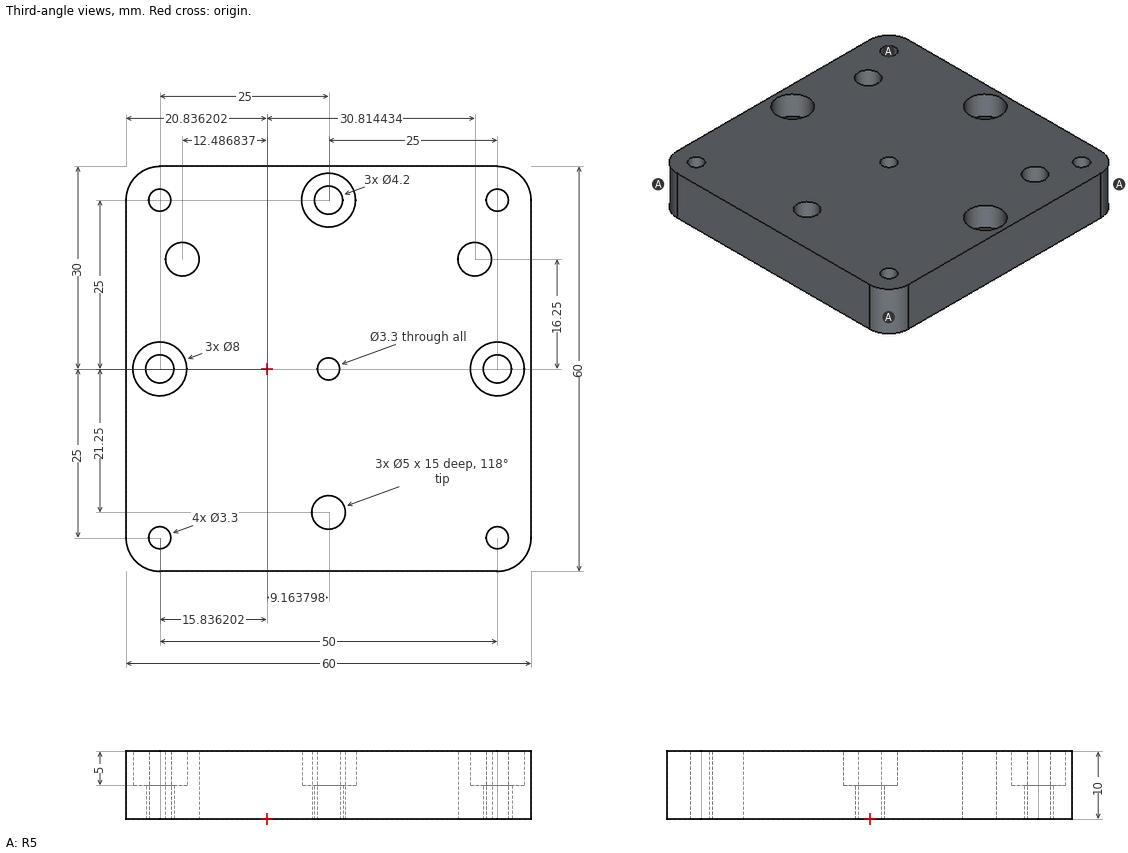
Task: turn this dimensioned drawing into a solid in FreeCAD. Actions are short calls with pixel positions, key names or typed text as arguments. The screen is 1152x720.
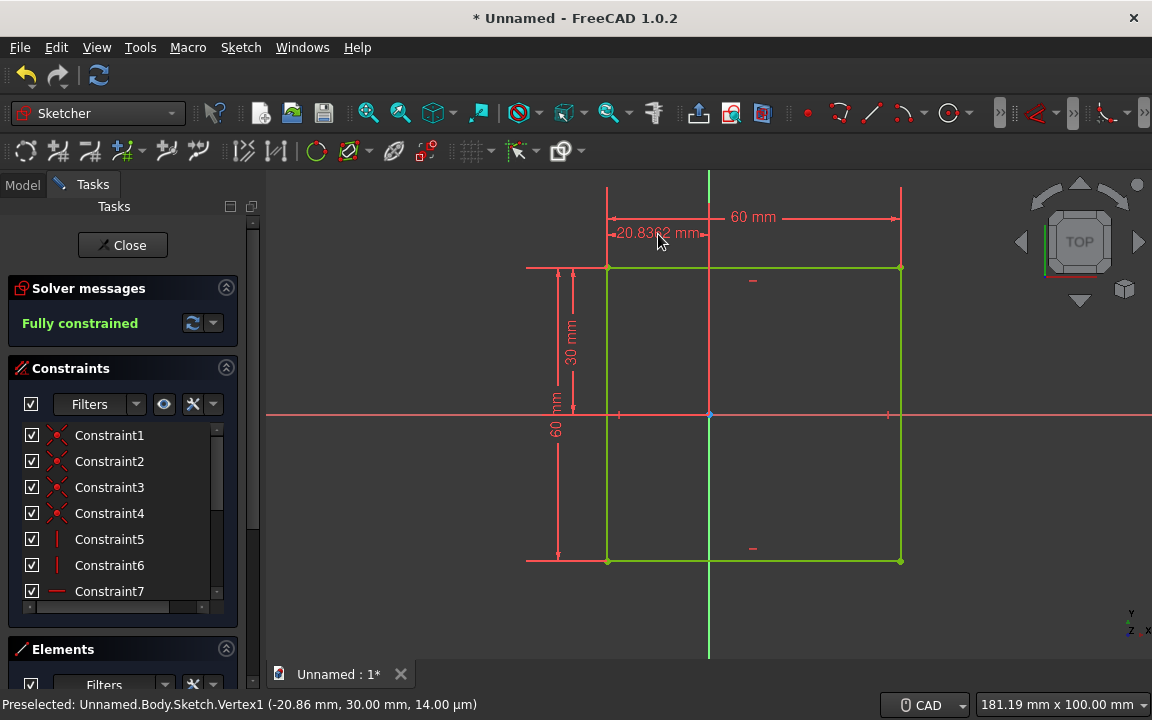
click(123, 245)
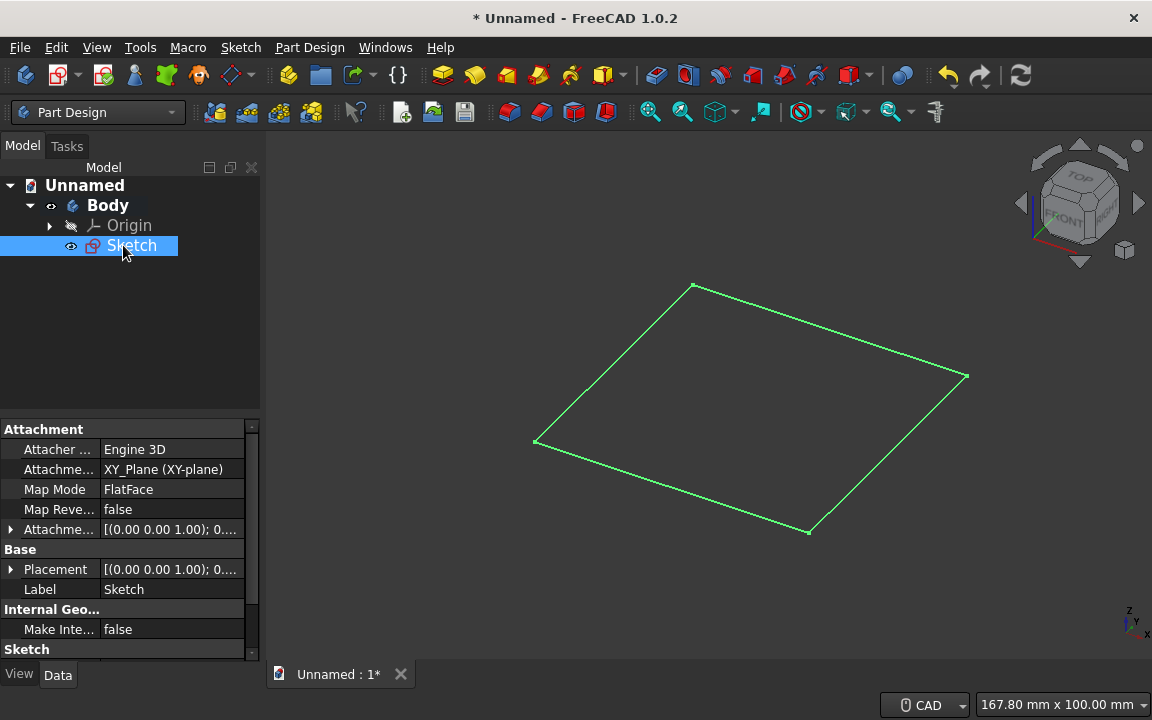
click(444, 76)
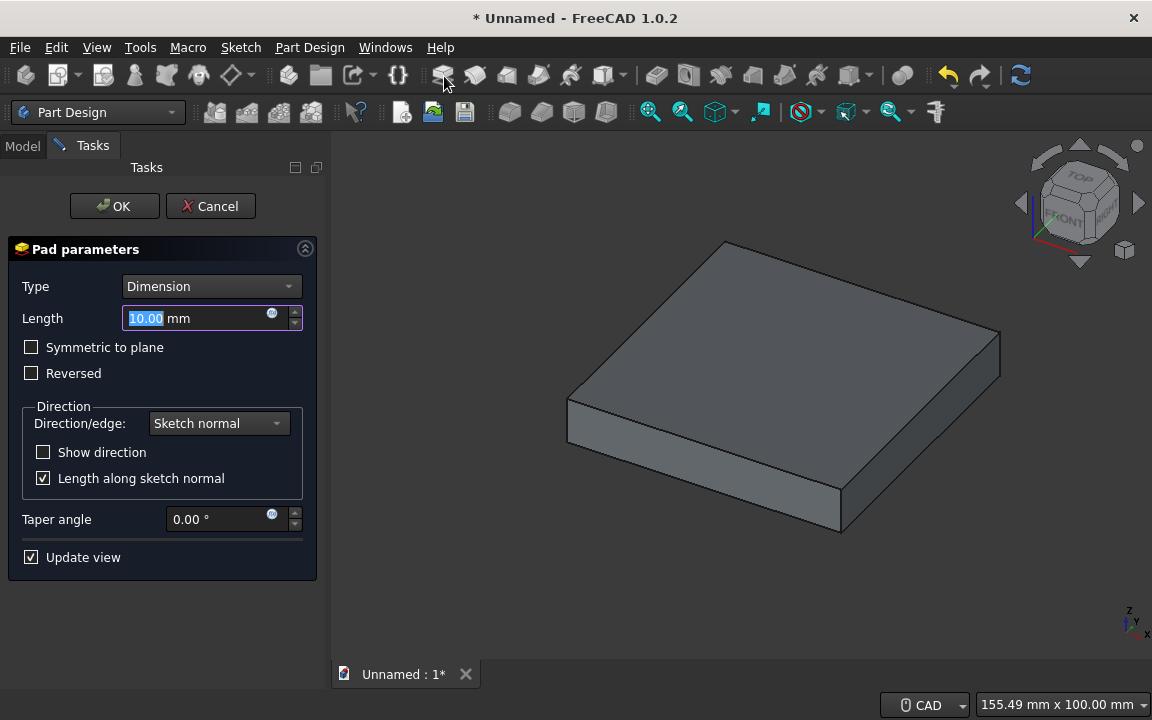
text(10)
key(Tab)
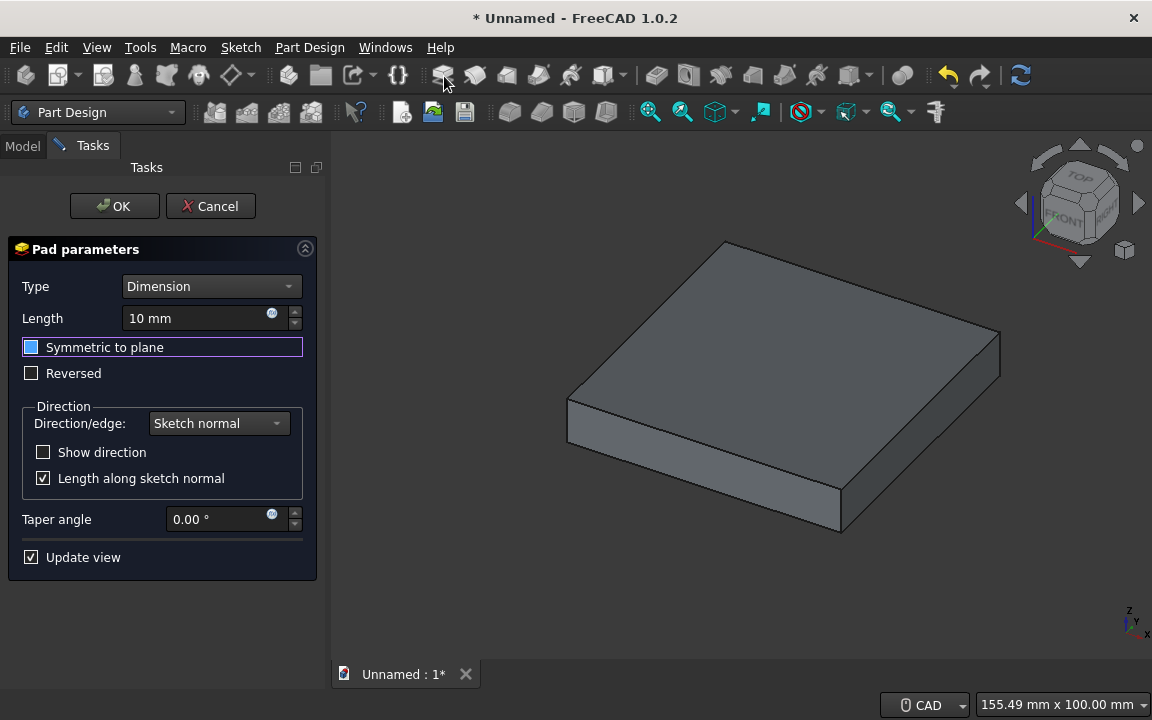
click(115, 206)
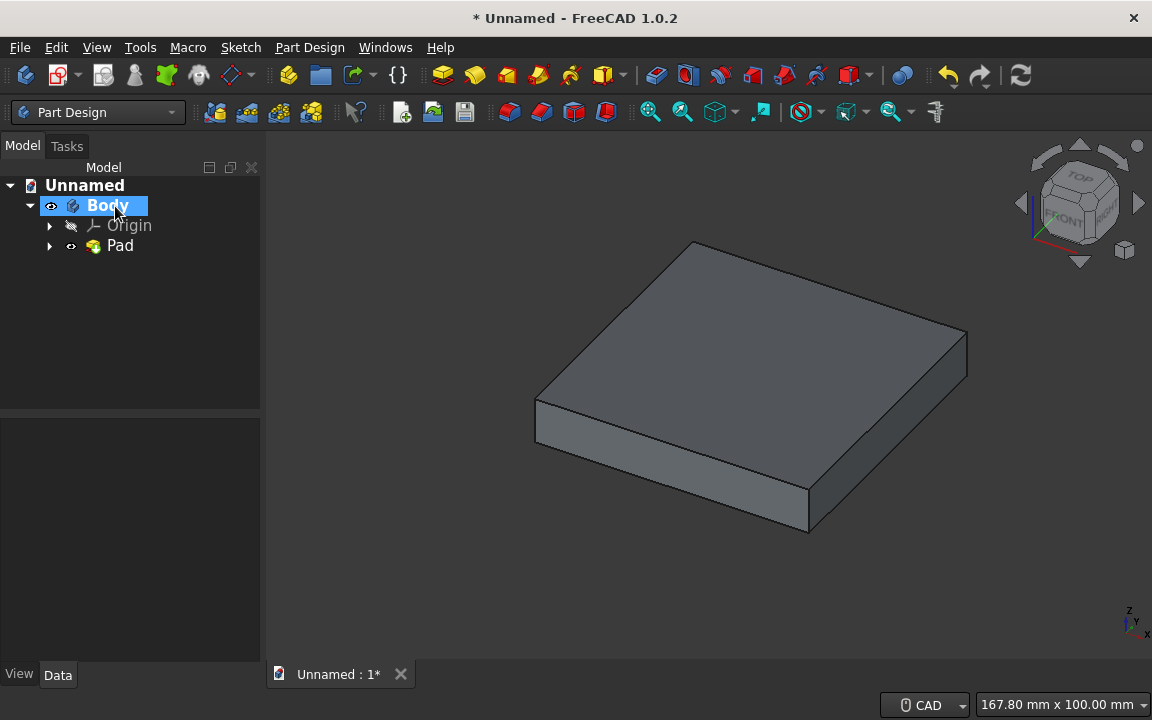
click(809, 510)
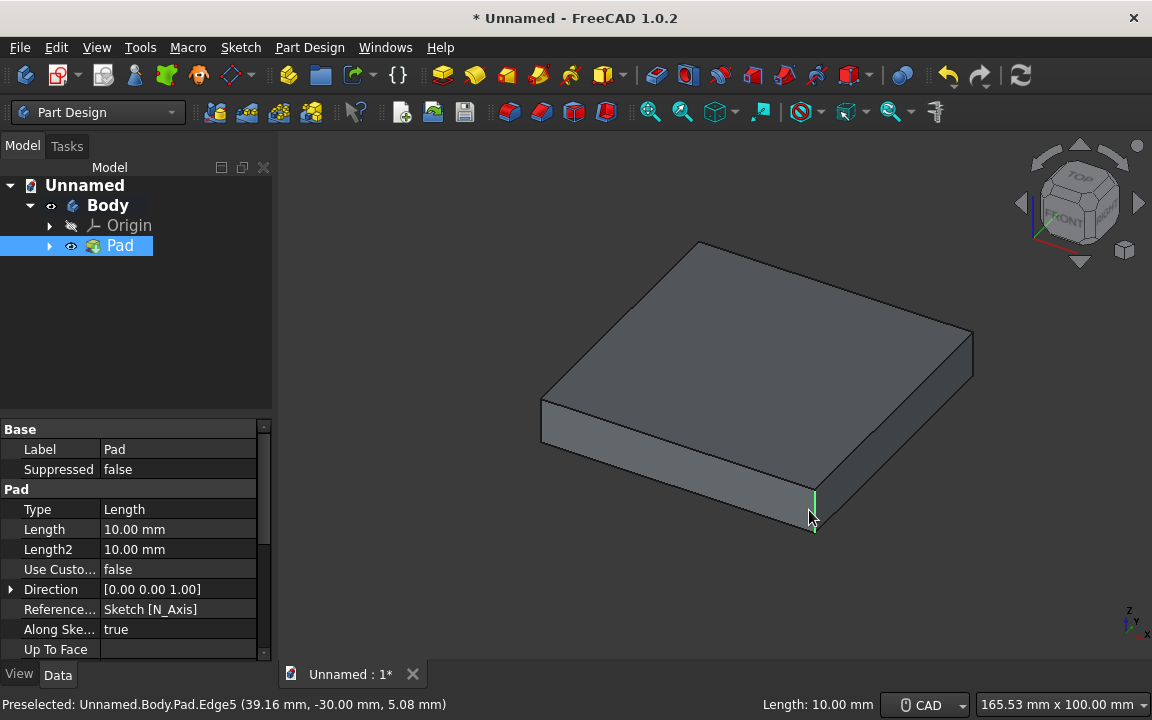
key(0)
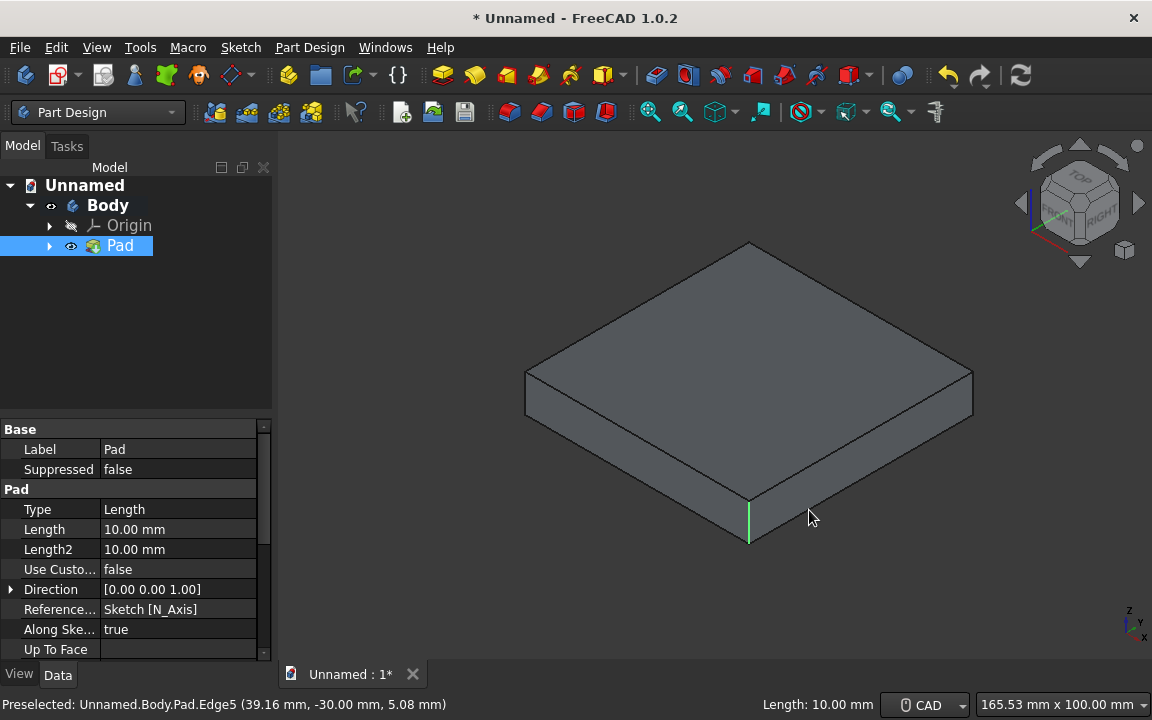
key(2)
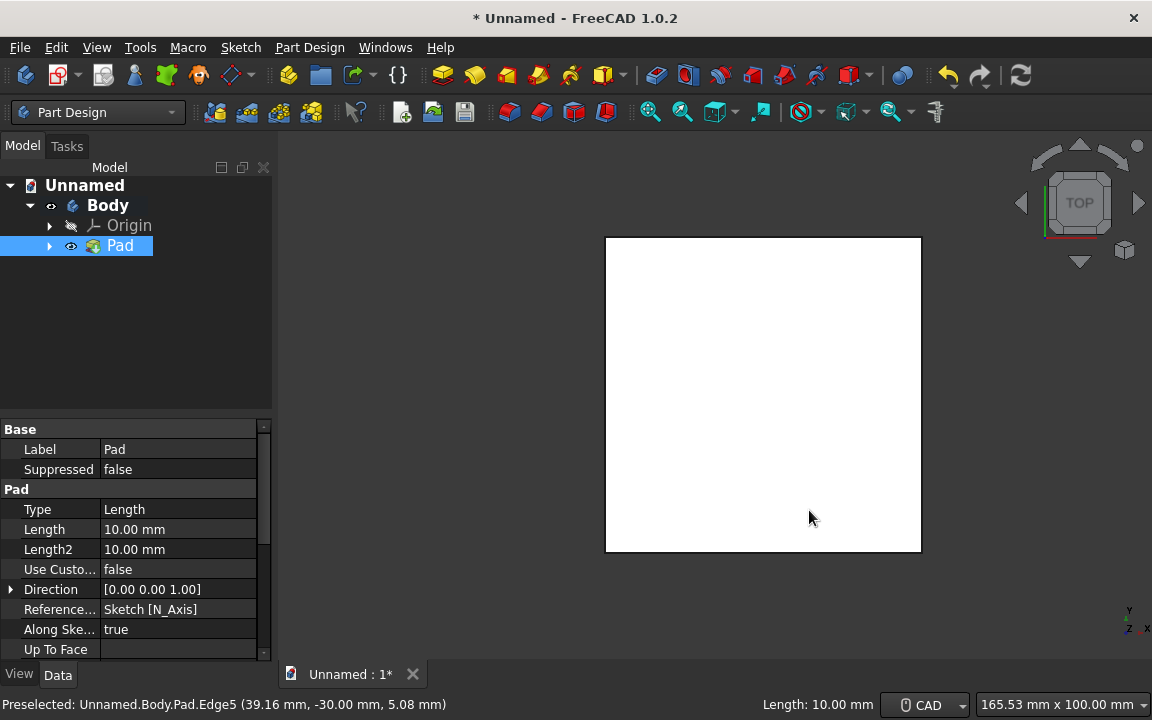
key(1)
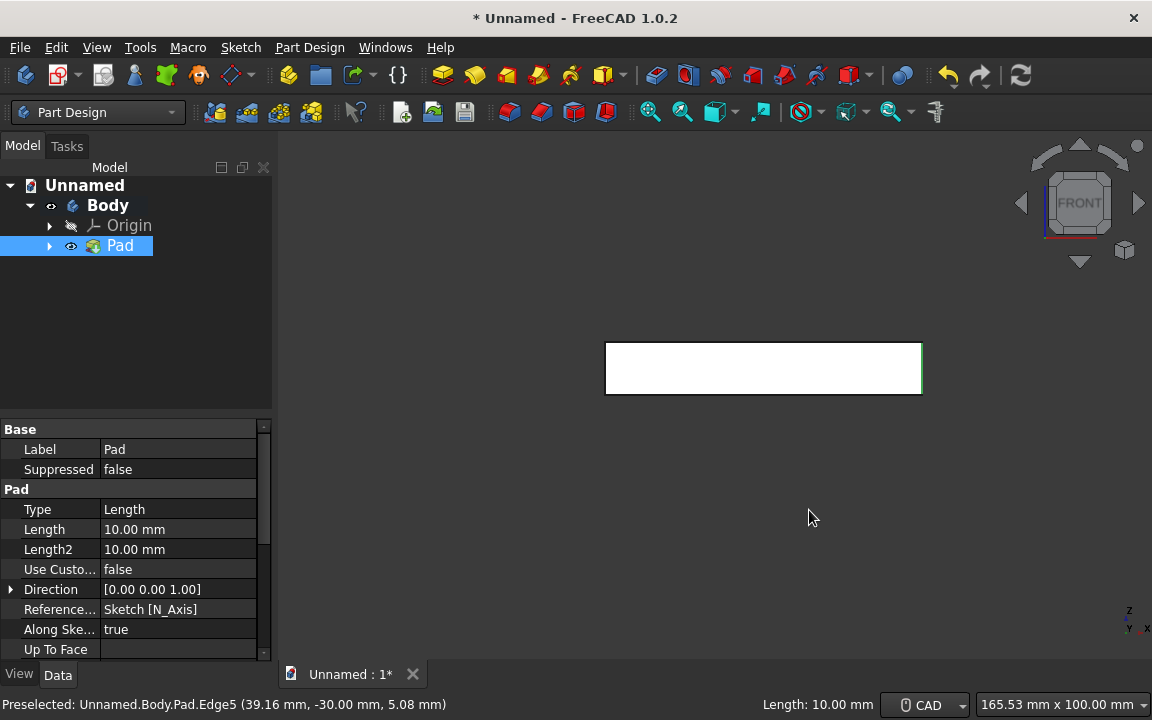
click(652, 112)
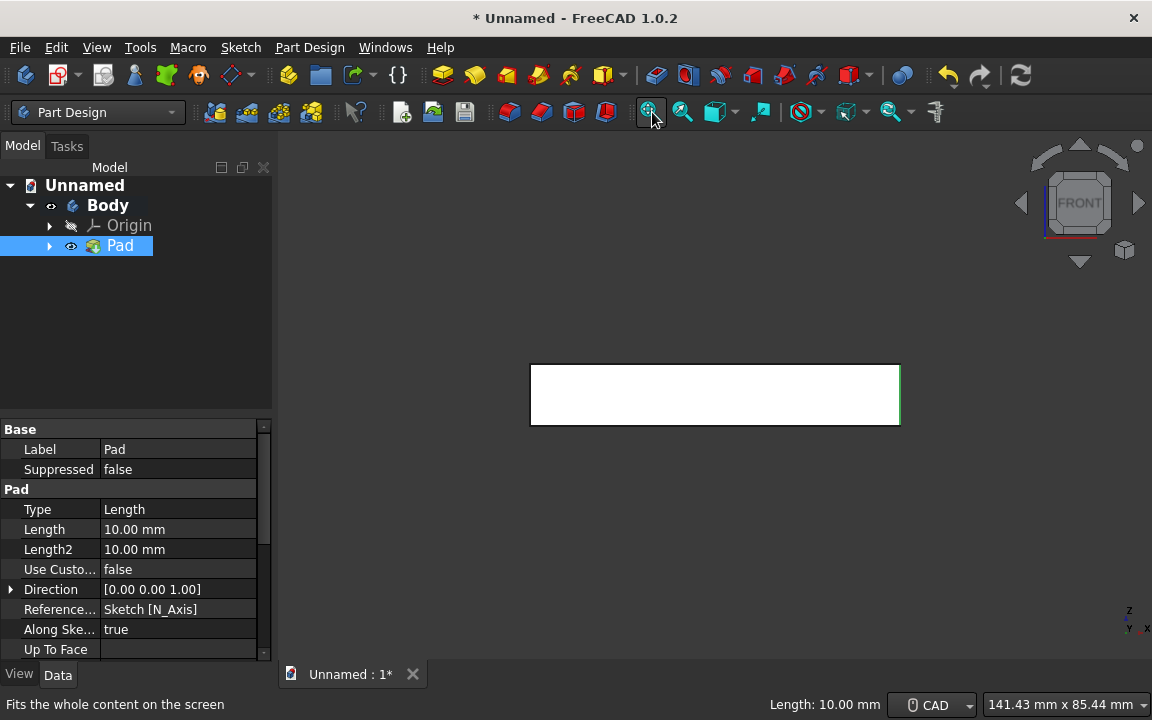
click(530, 394, ctrl)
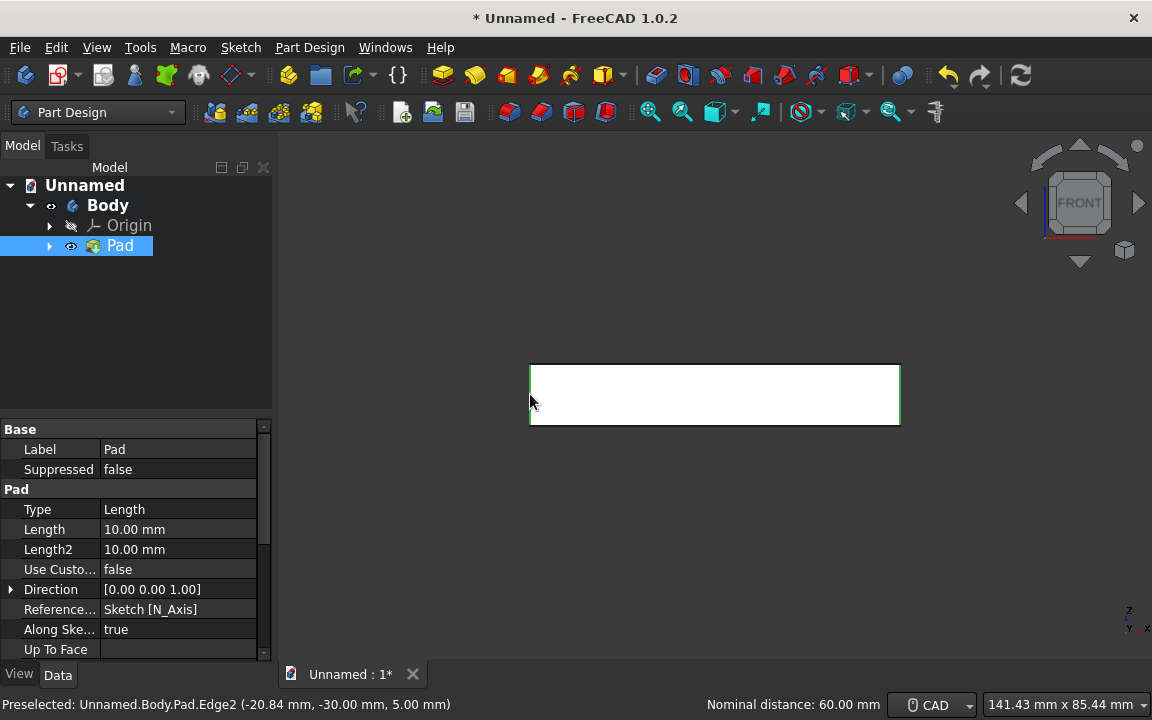
key(3)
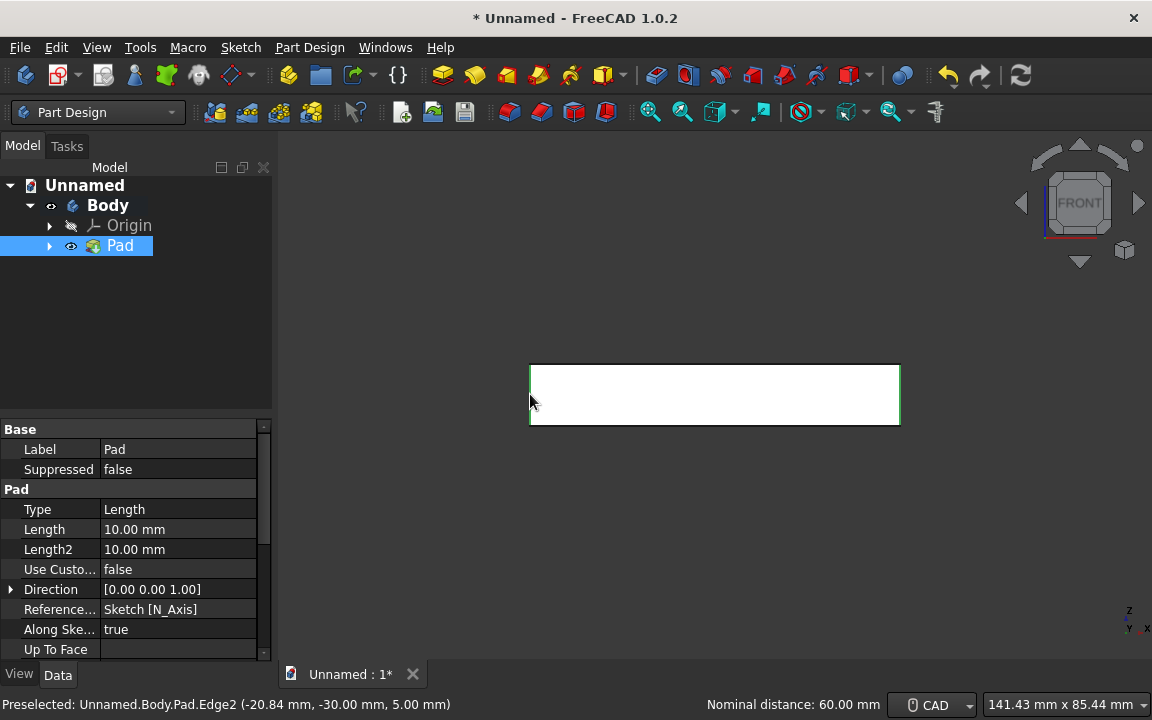
click(652, 112)